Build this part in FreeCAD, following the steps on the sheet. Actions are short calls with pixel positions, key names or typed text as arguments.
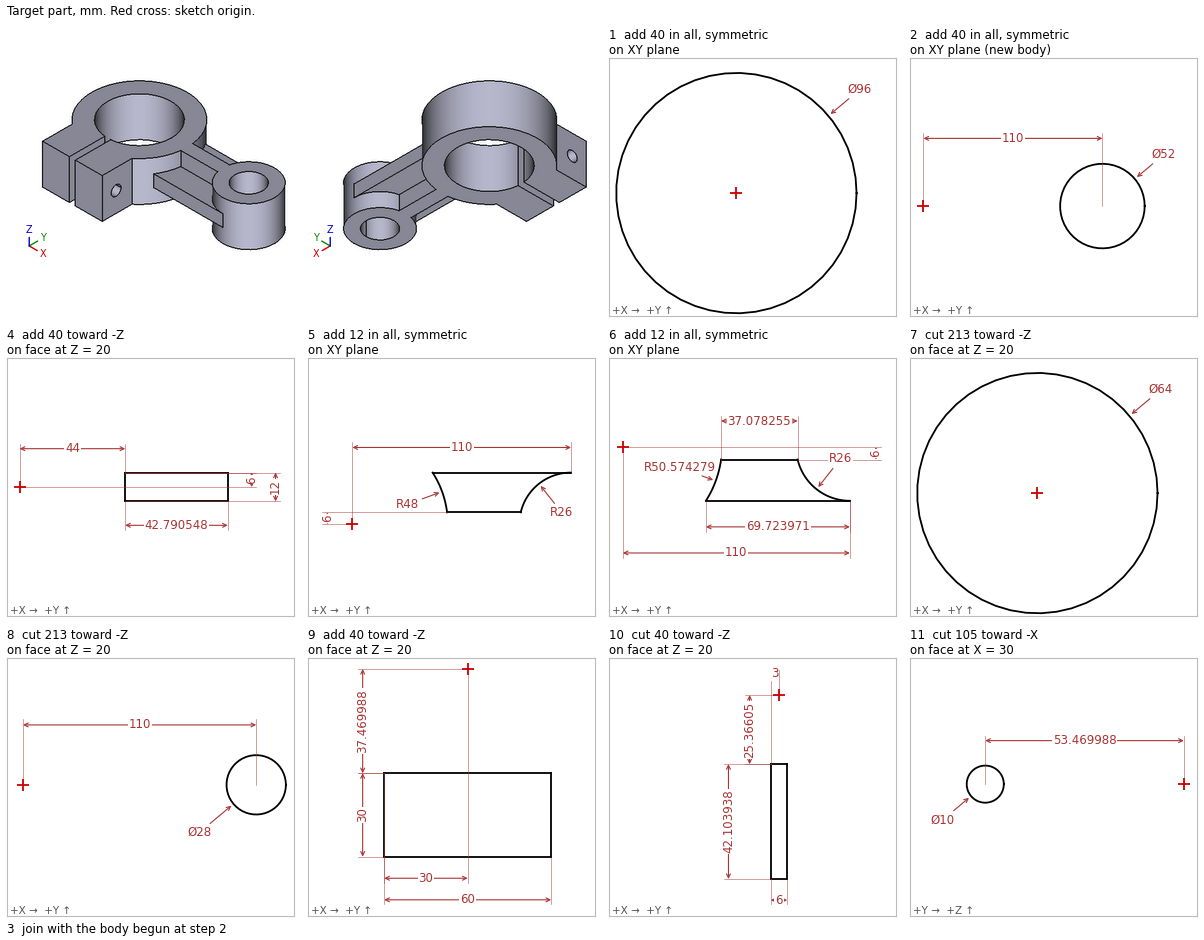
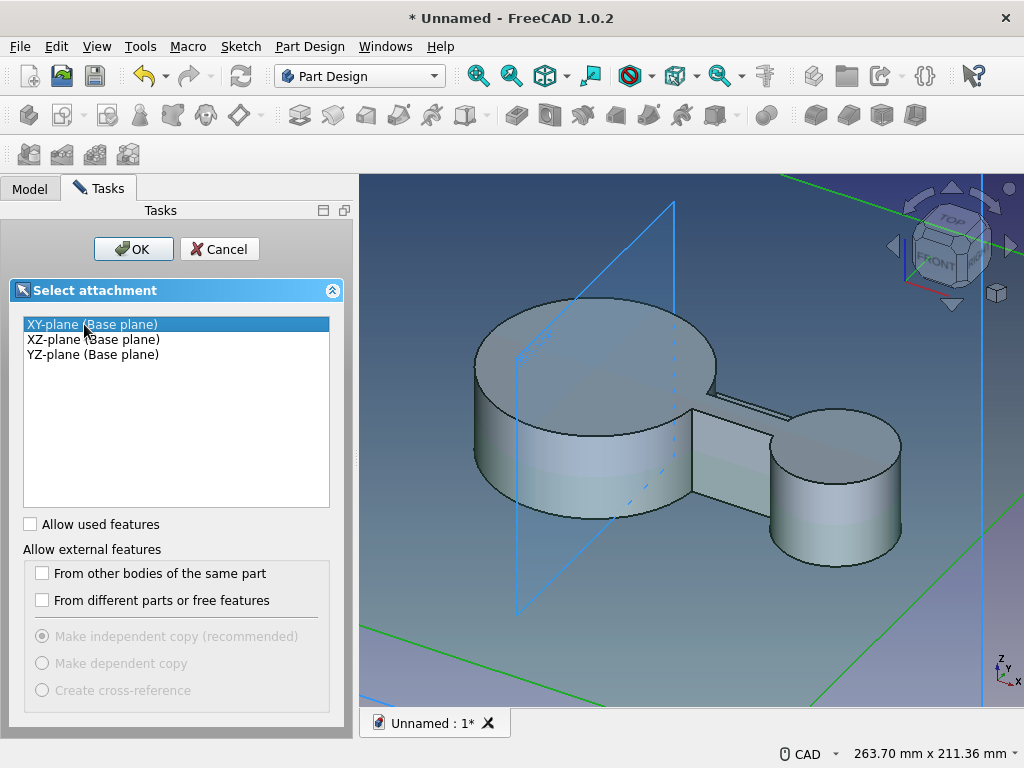
click(134, 249)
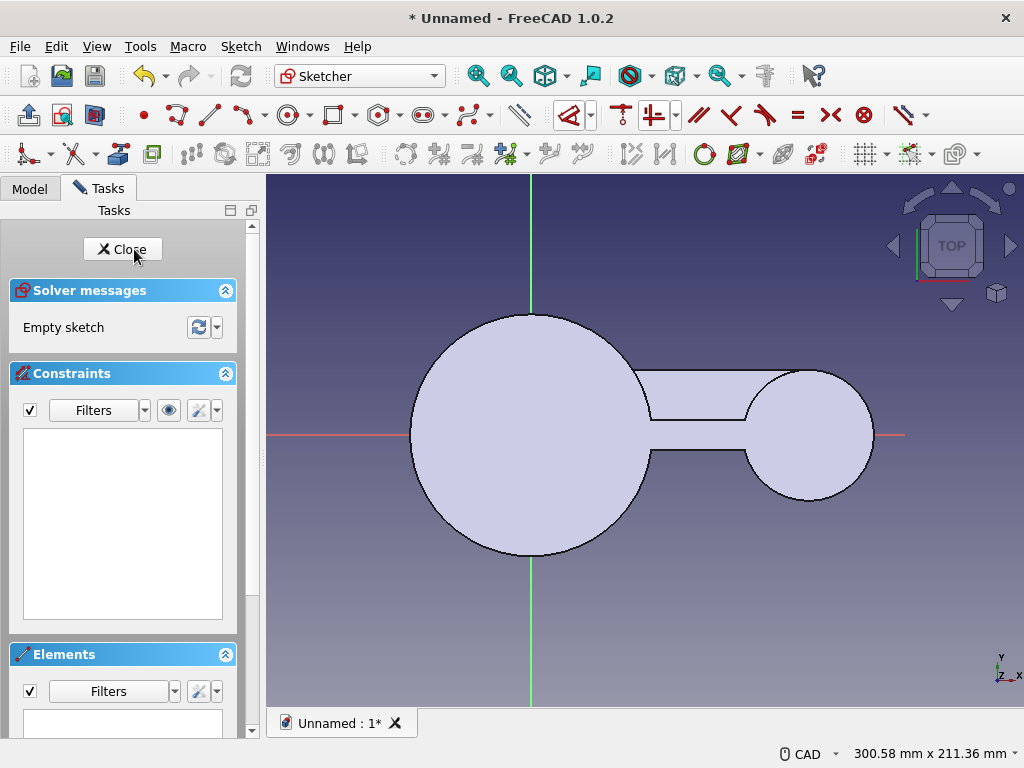
click(95, 116)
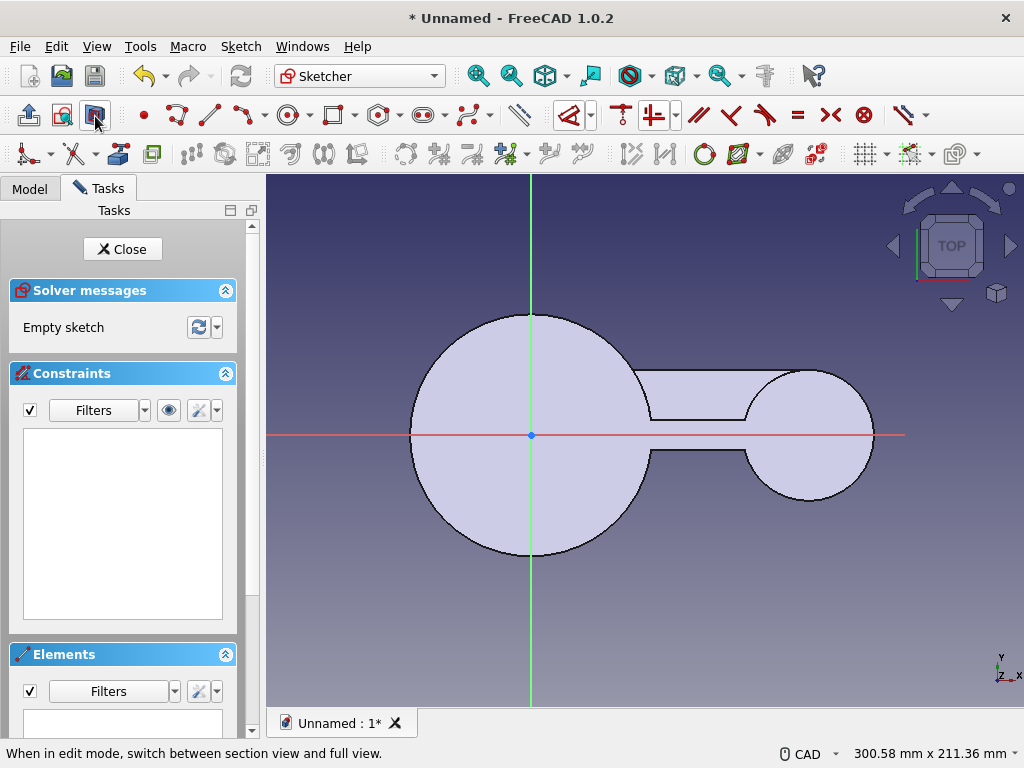
scroll(859, 524, up, 2)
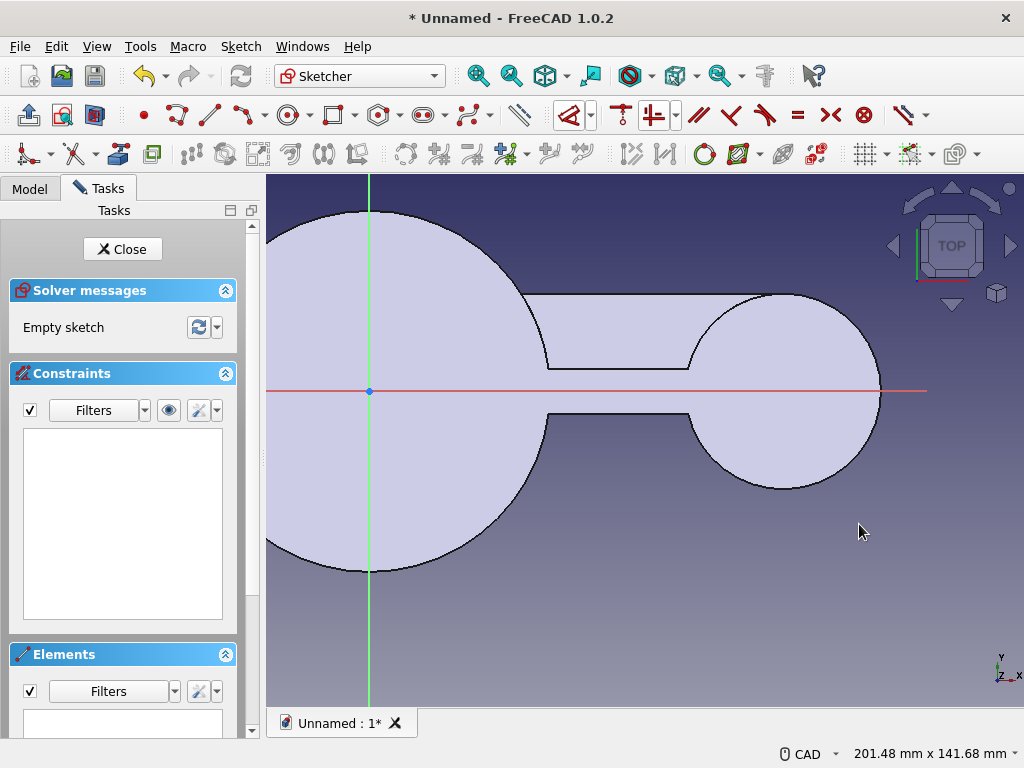
click(210, 116)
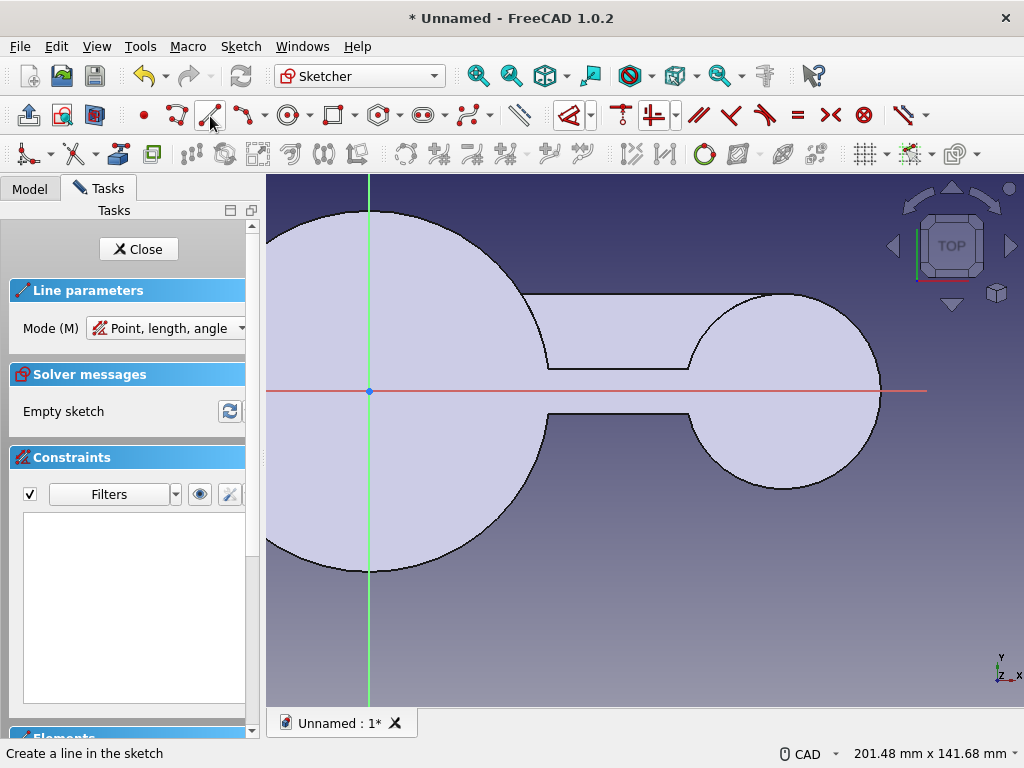
click(521, 489)
click(783, 489)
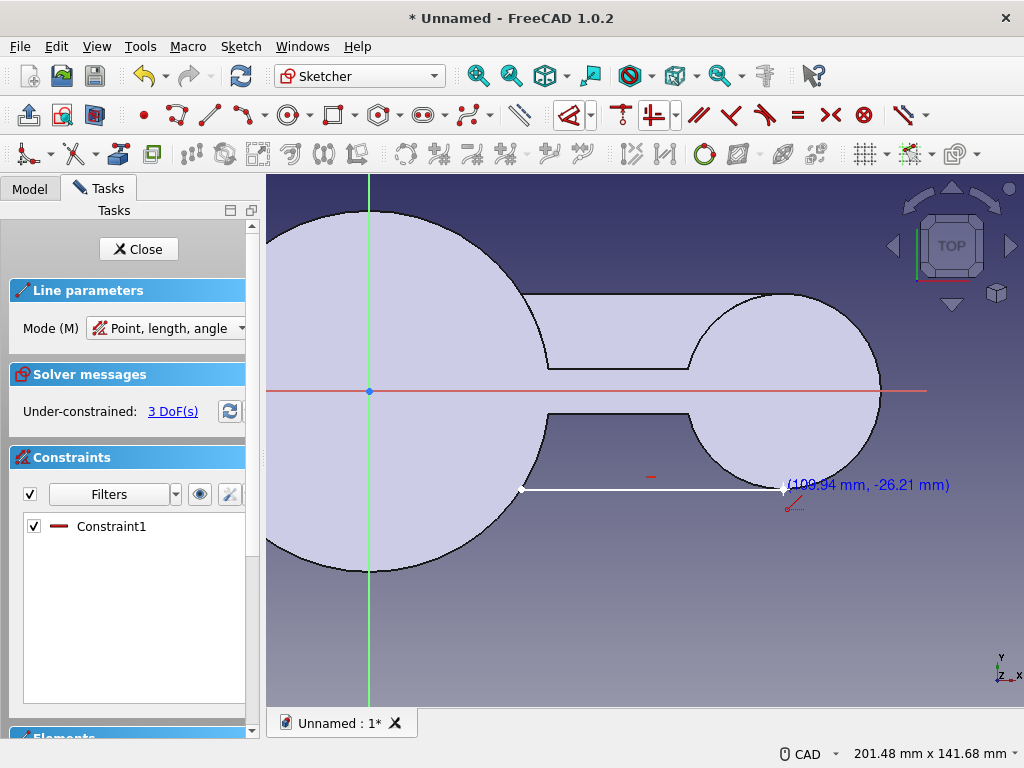
click(688, 414)
click(549, 414)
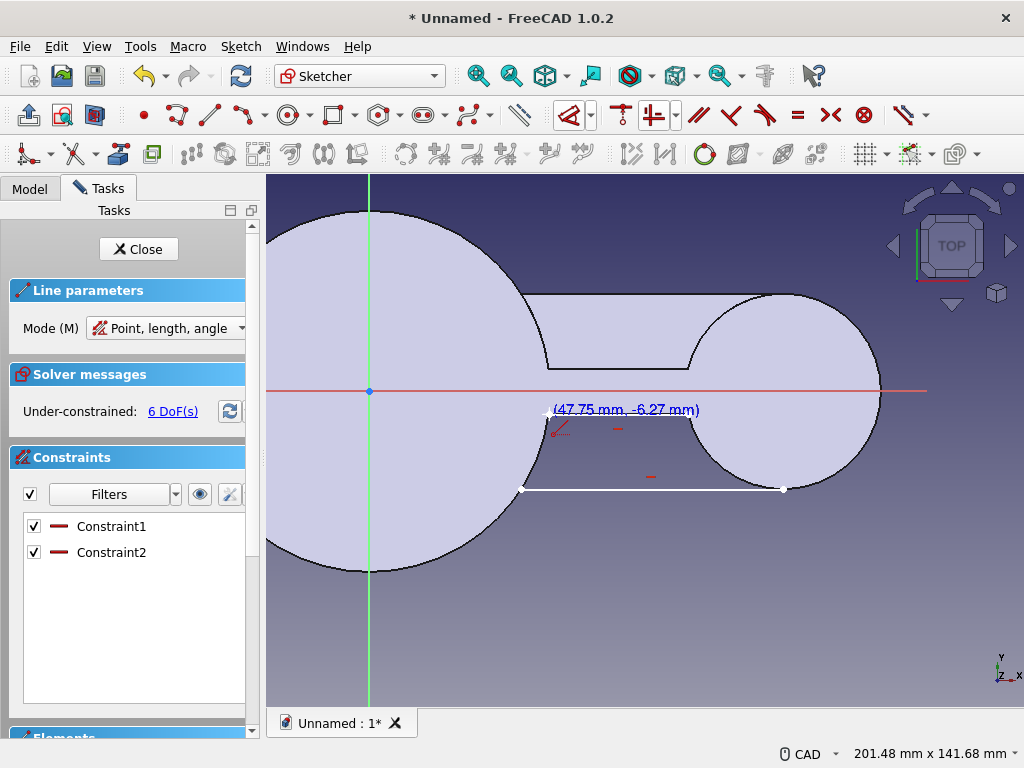
click(242, 116)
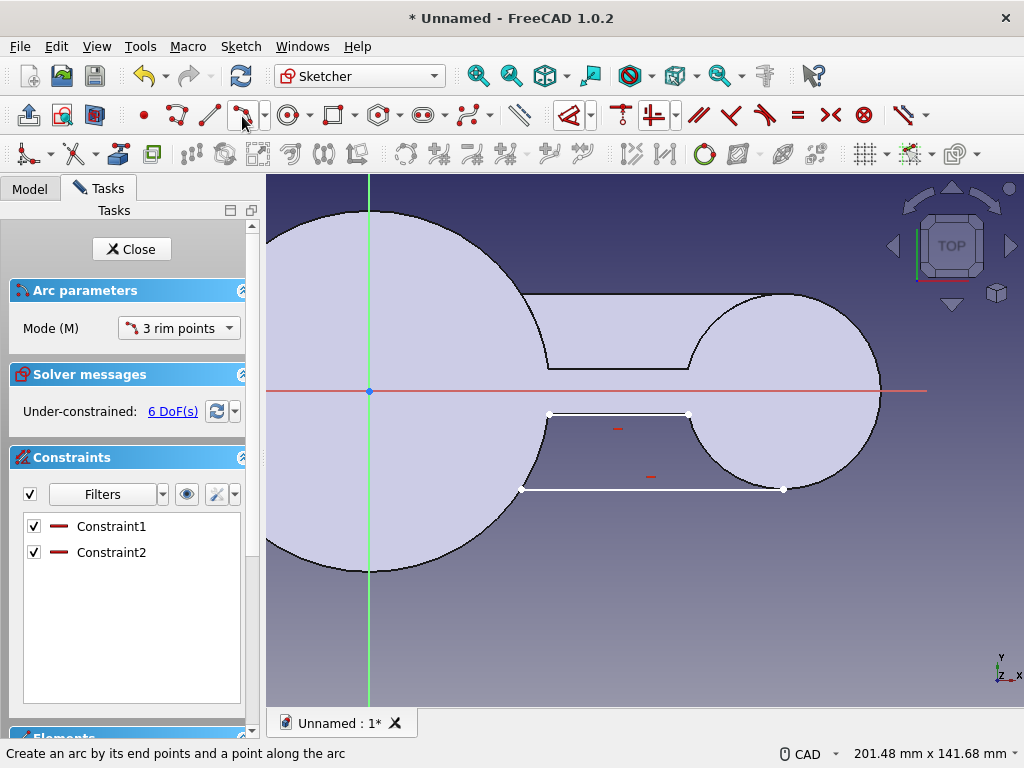
click(783, 490)
click(688, 415)
click(723, 468)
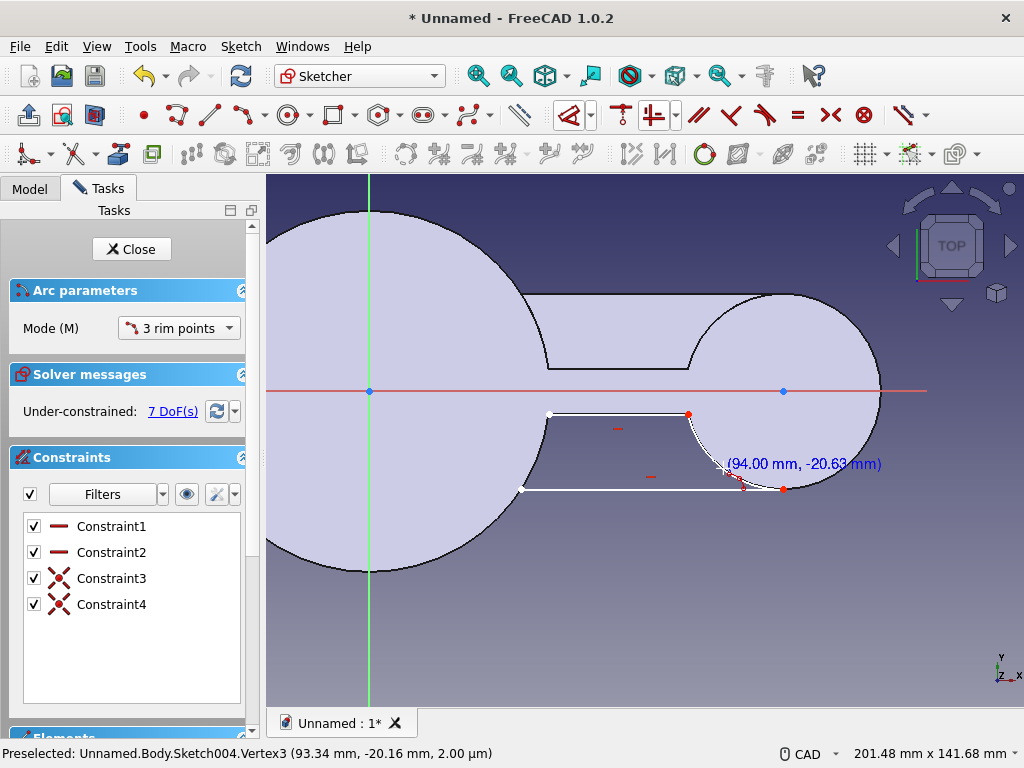
click(549, 415)
click(521, 490)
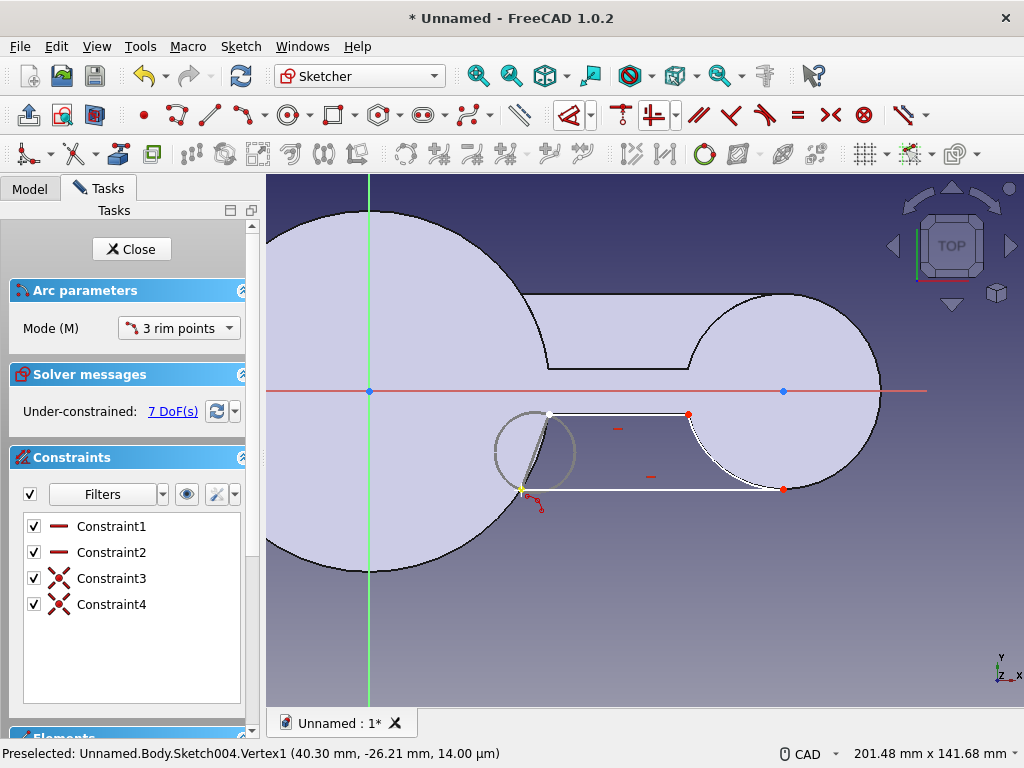
scroll(539, 453, up, 7)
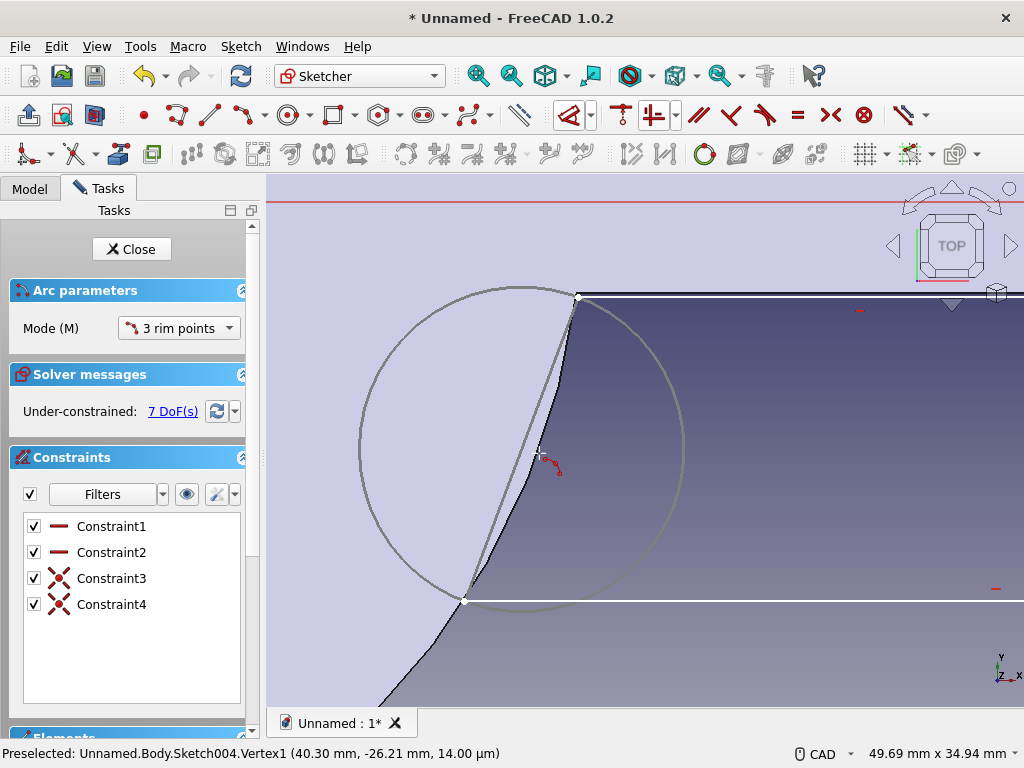
click(537, 452)
key(Escape)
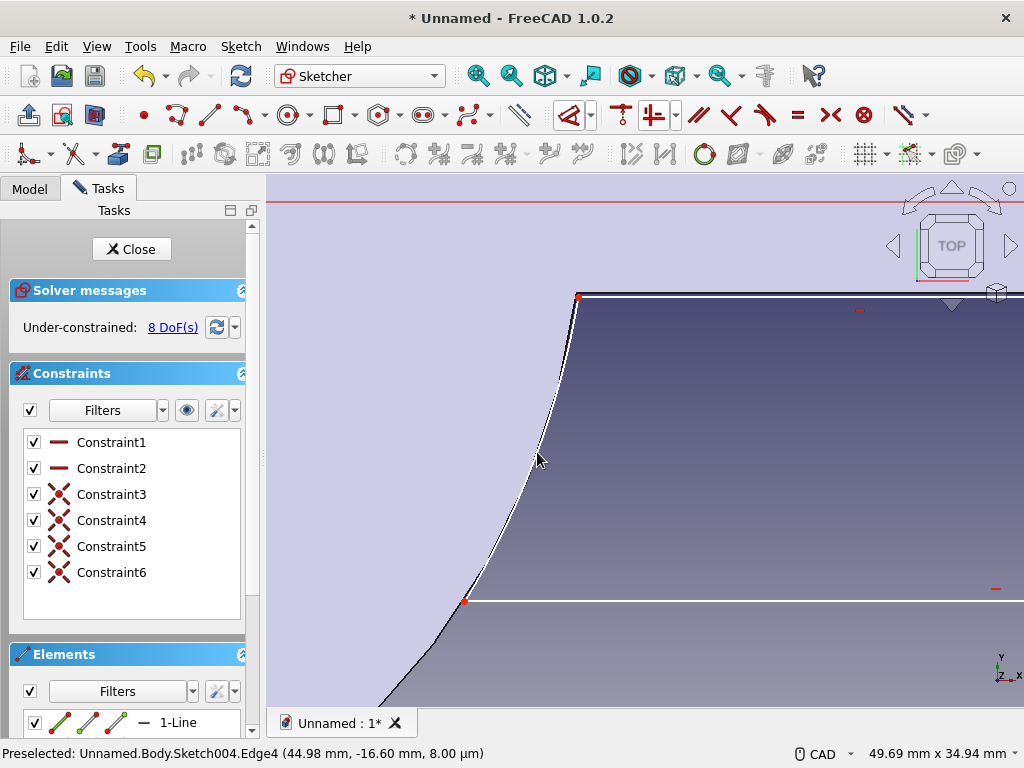
scroll(540, 454, down, 7)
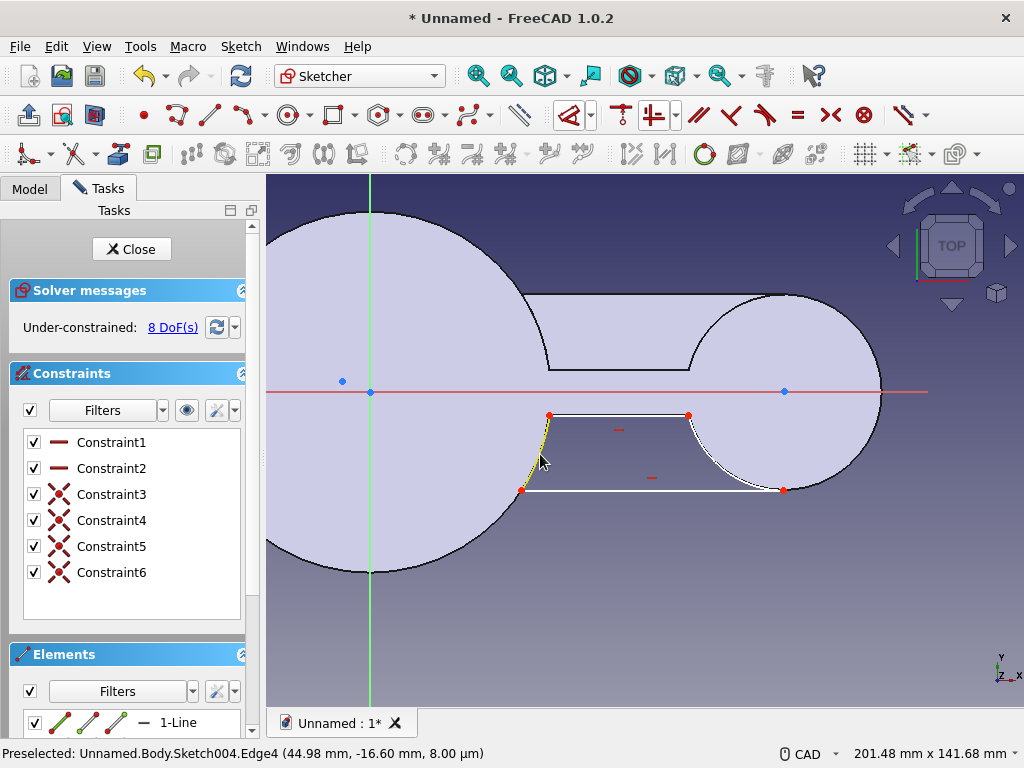
click(600, 491)